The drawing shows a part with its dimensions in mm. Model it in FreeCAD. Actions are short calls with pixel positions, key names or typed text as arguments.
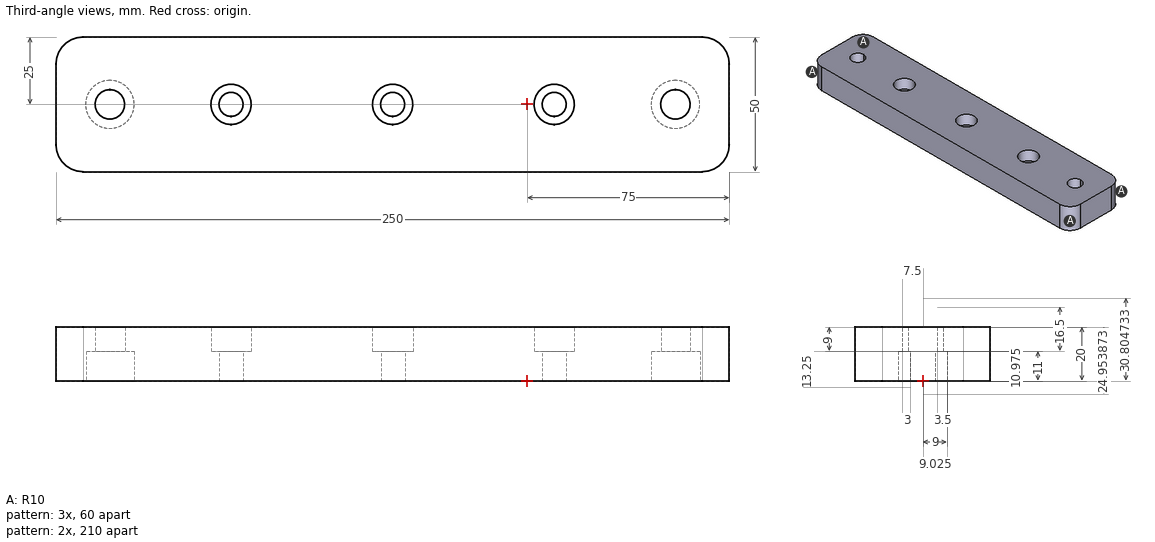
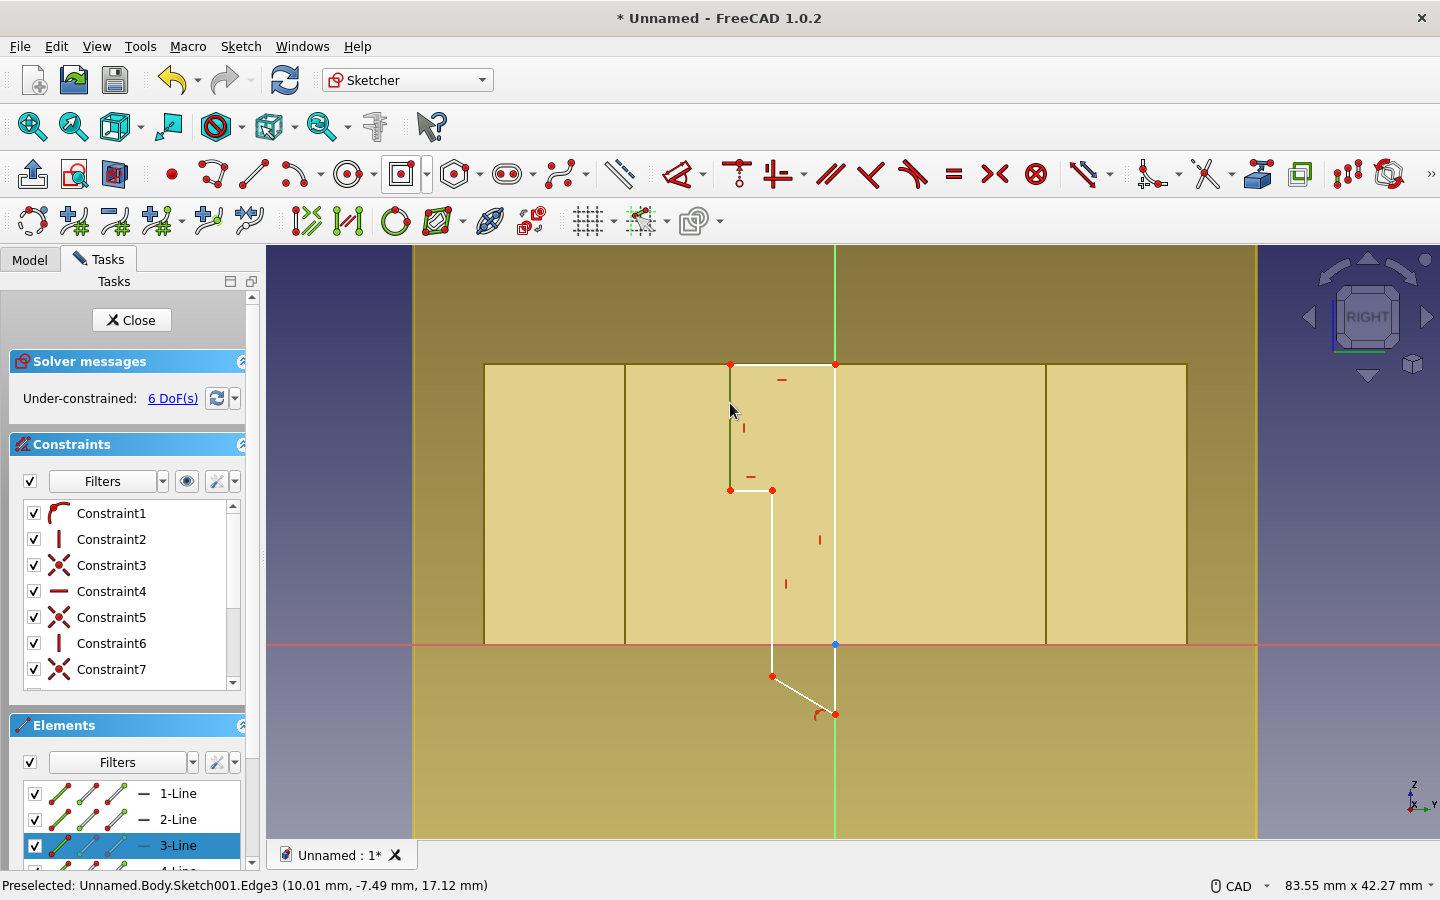
key(i)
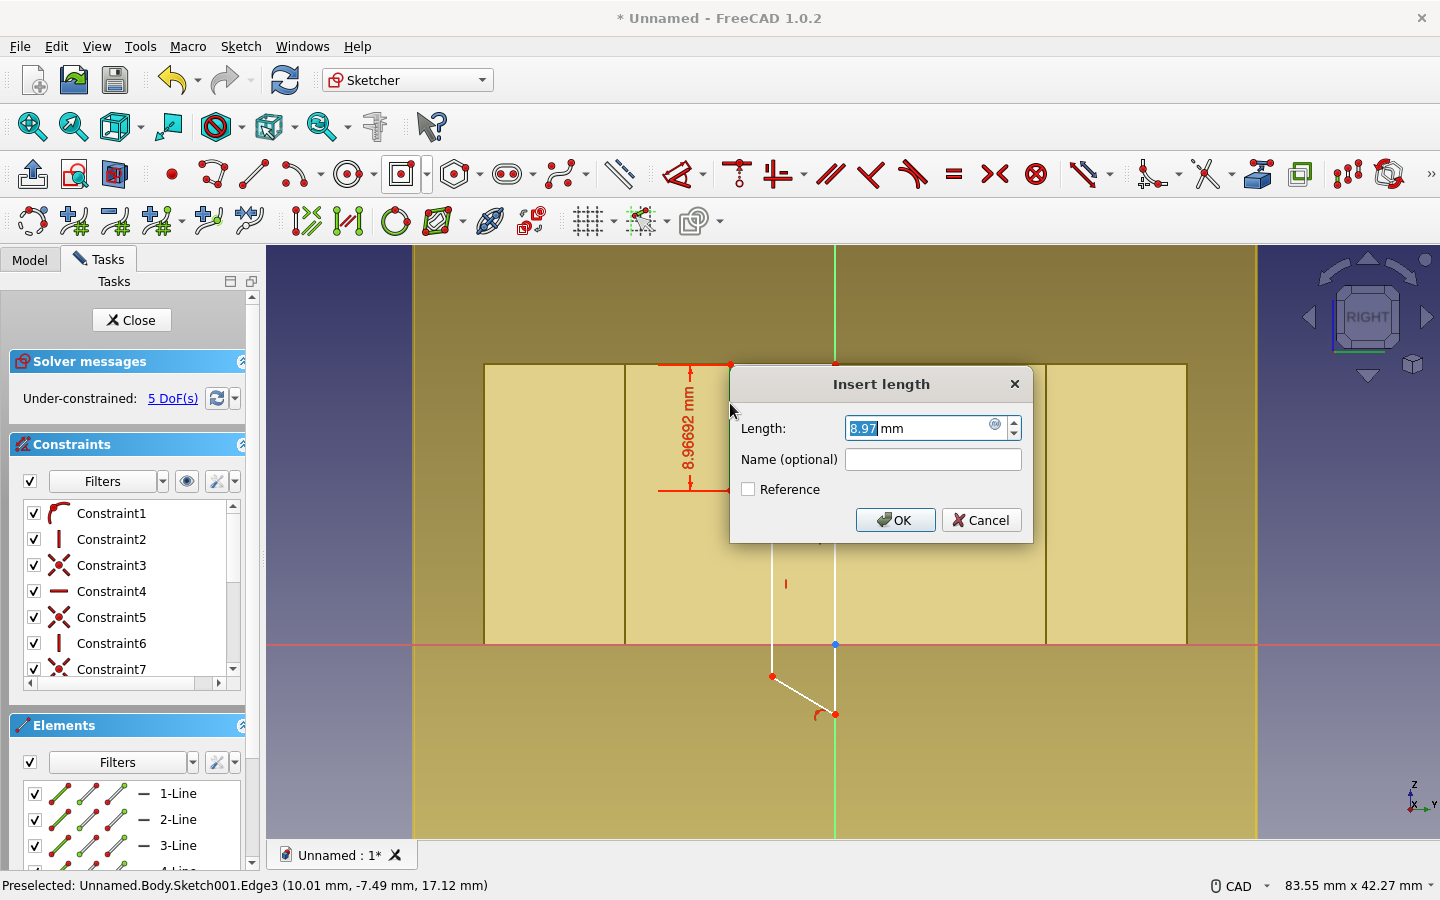
text(9)
key(Return)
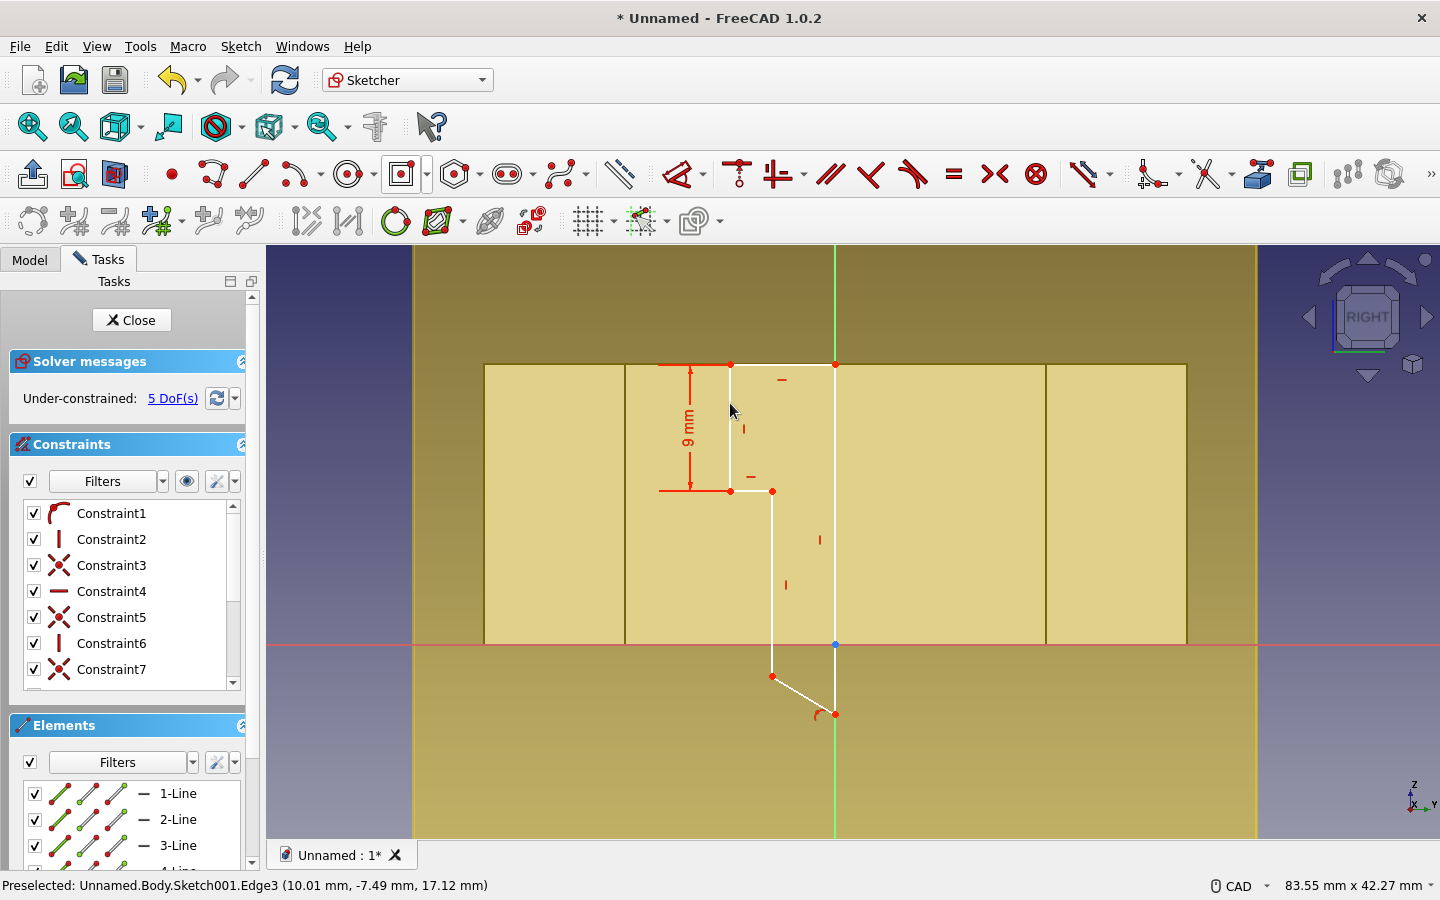
click(743, 491)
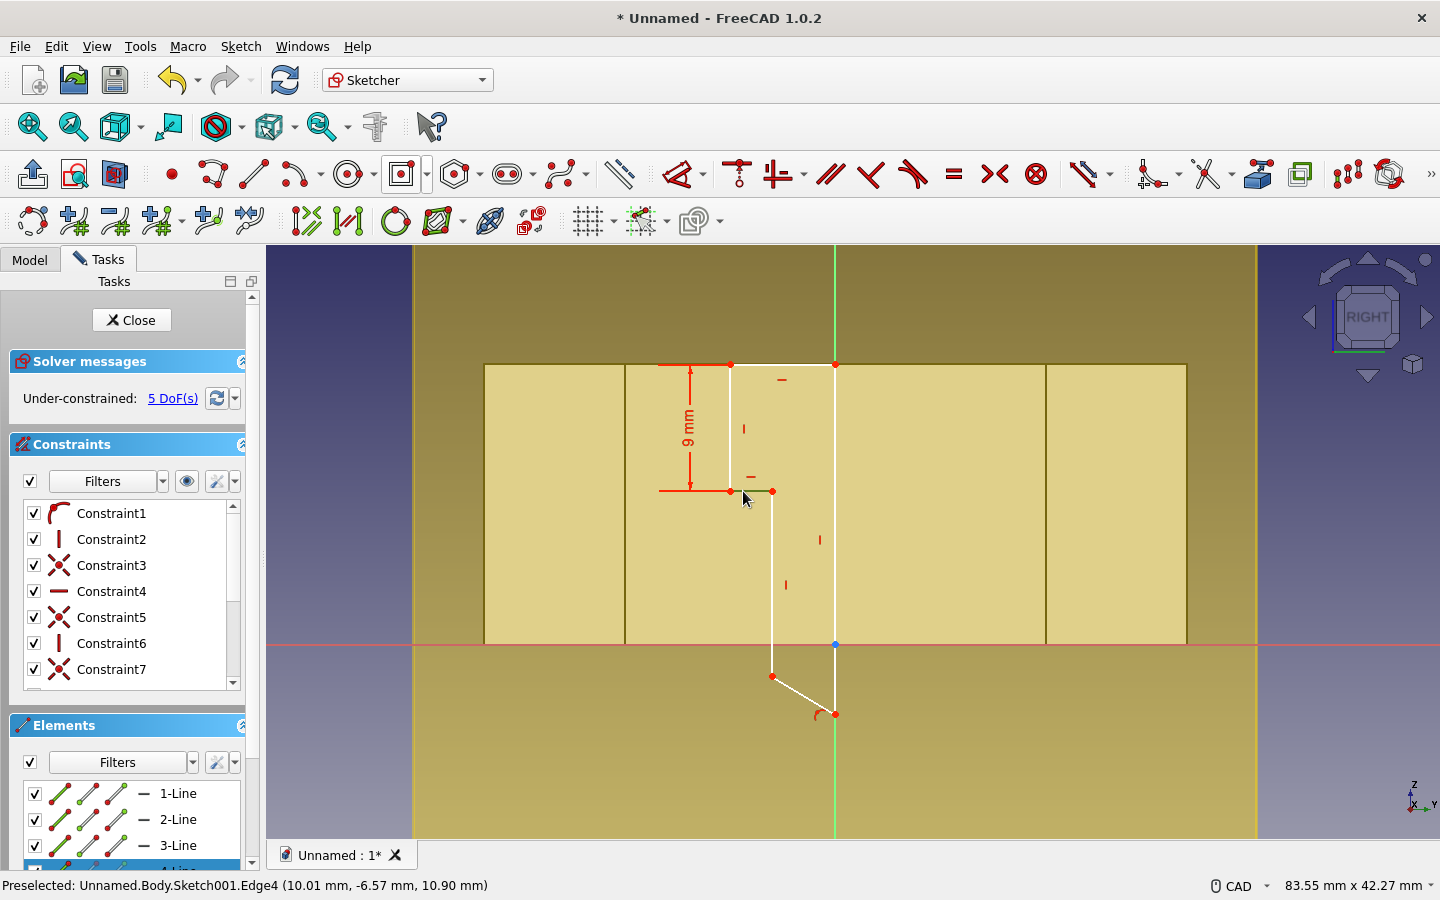
key(l)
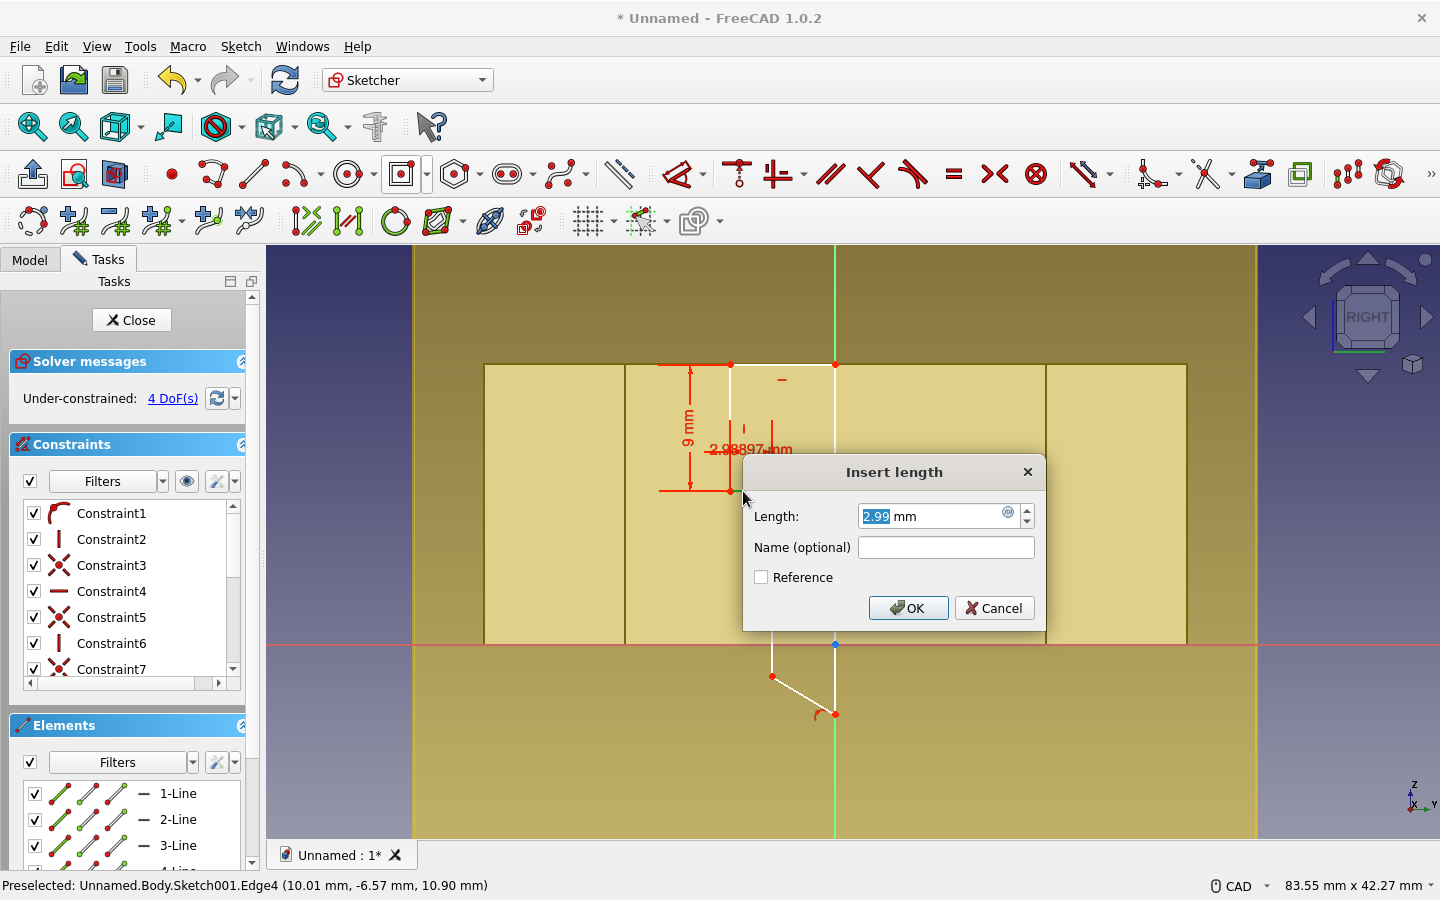
text(3)
key(Return)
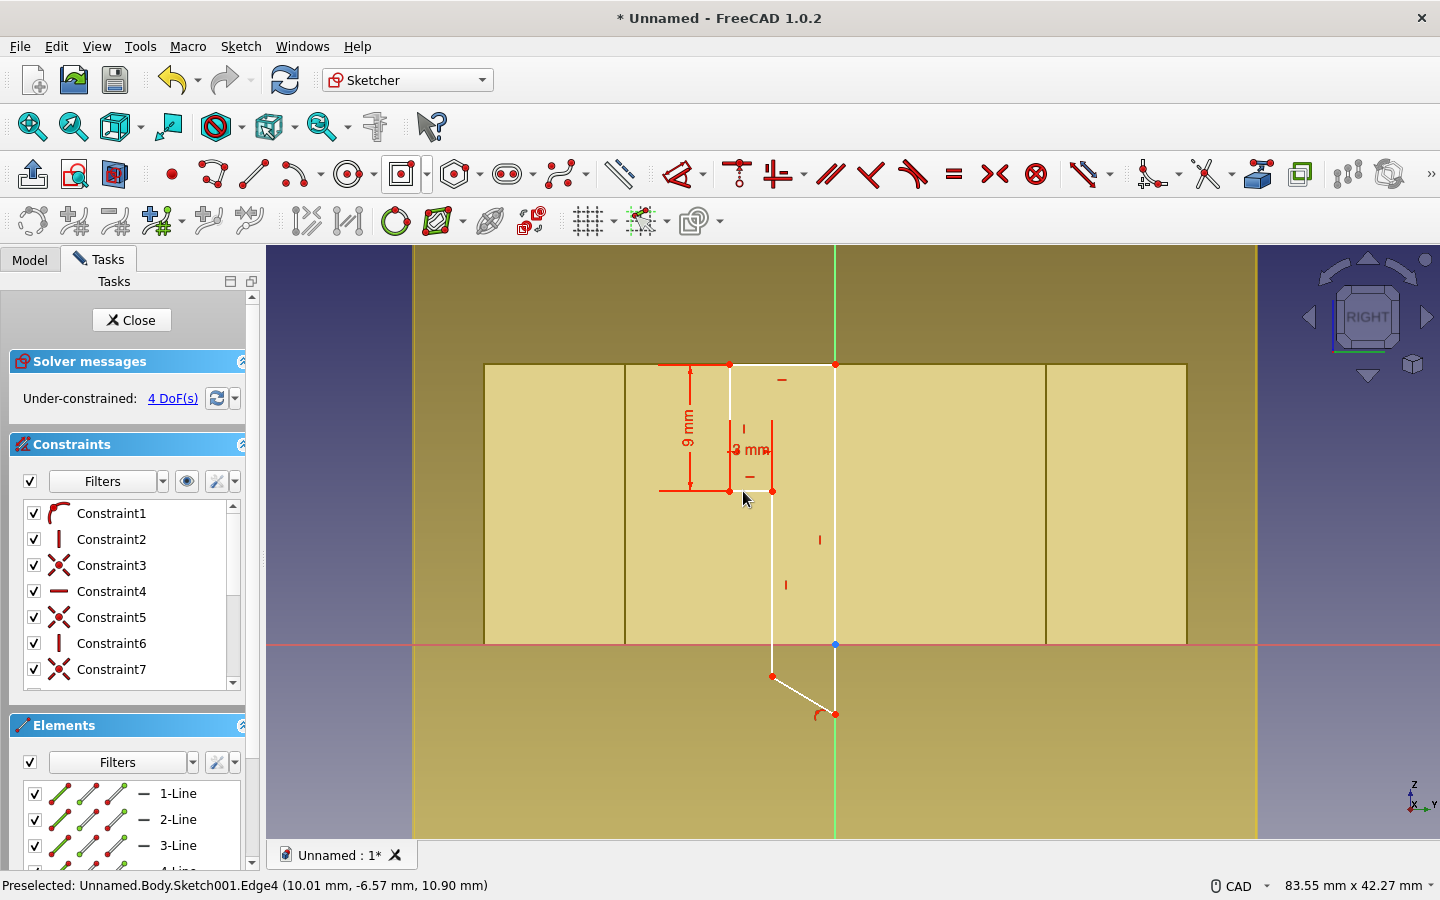
click(804, 365)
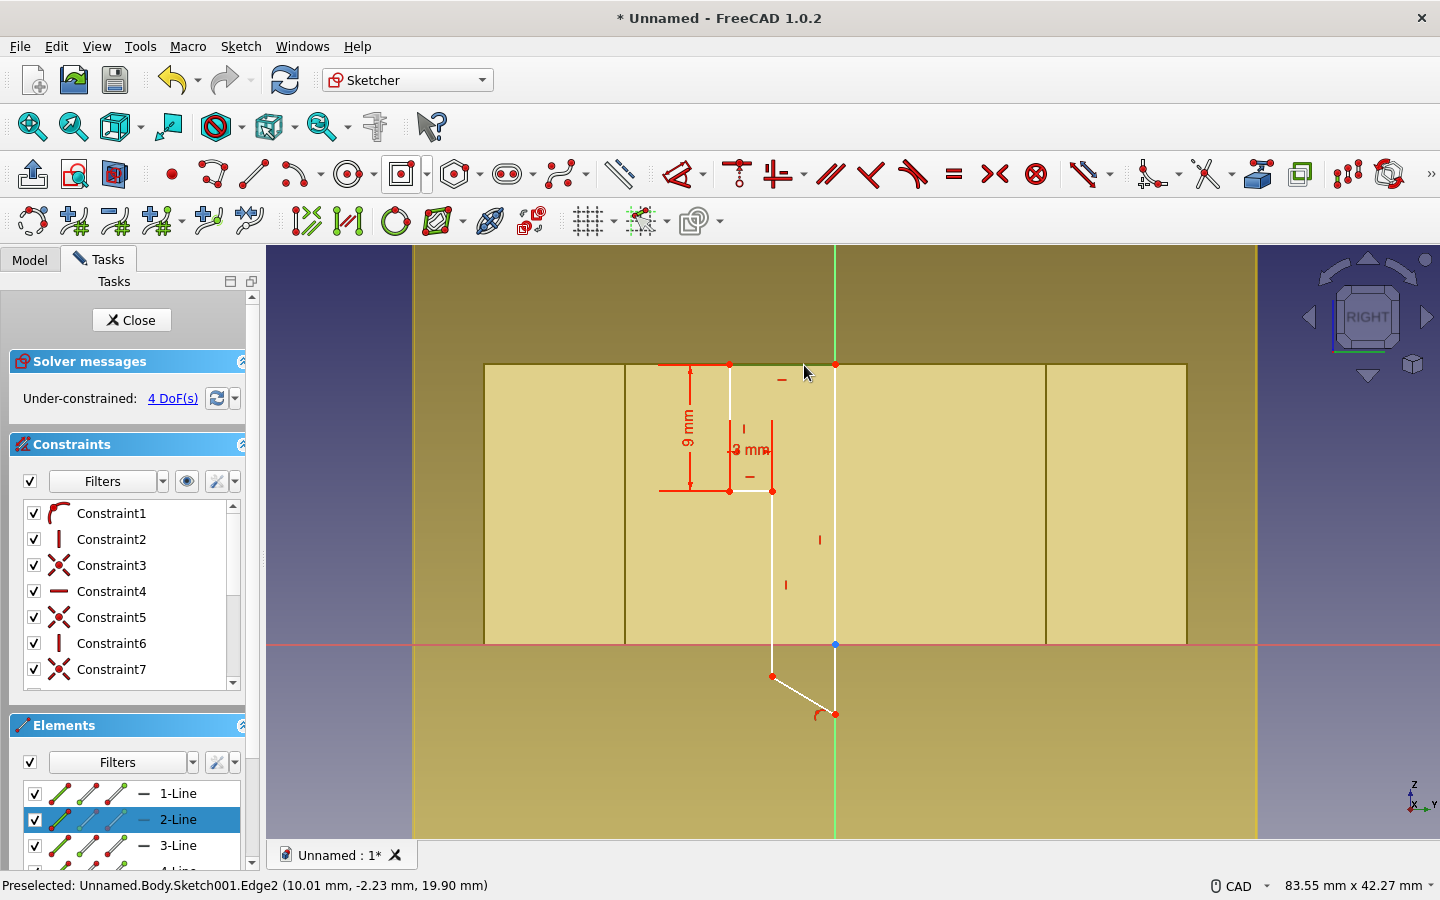
key(l)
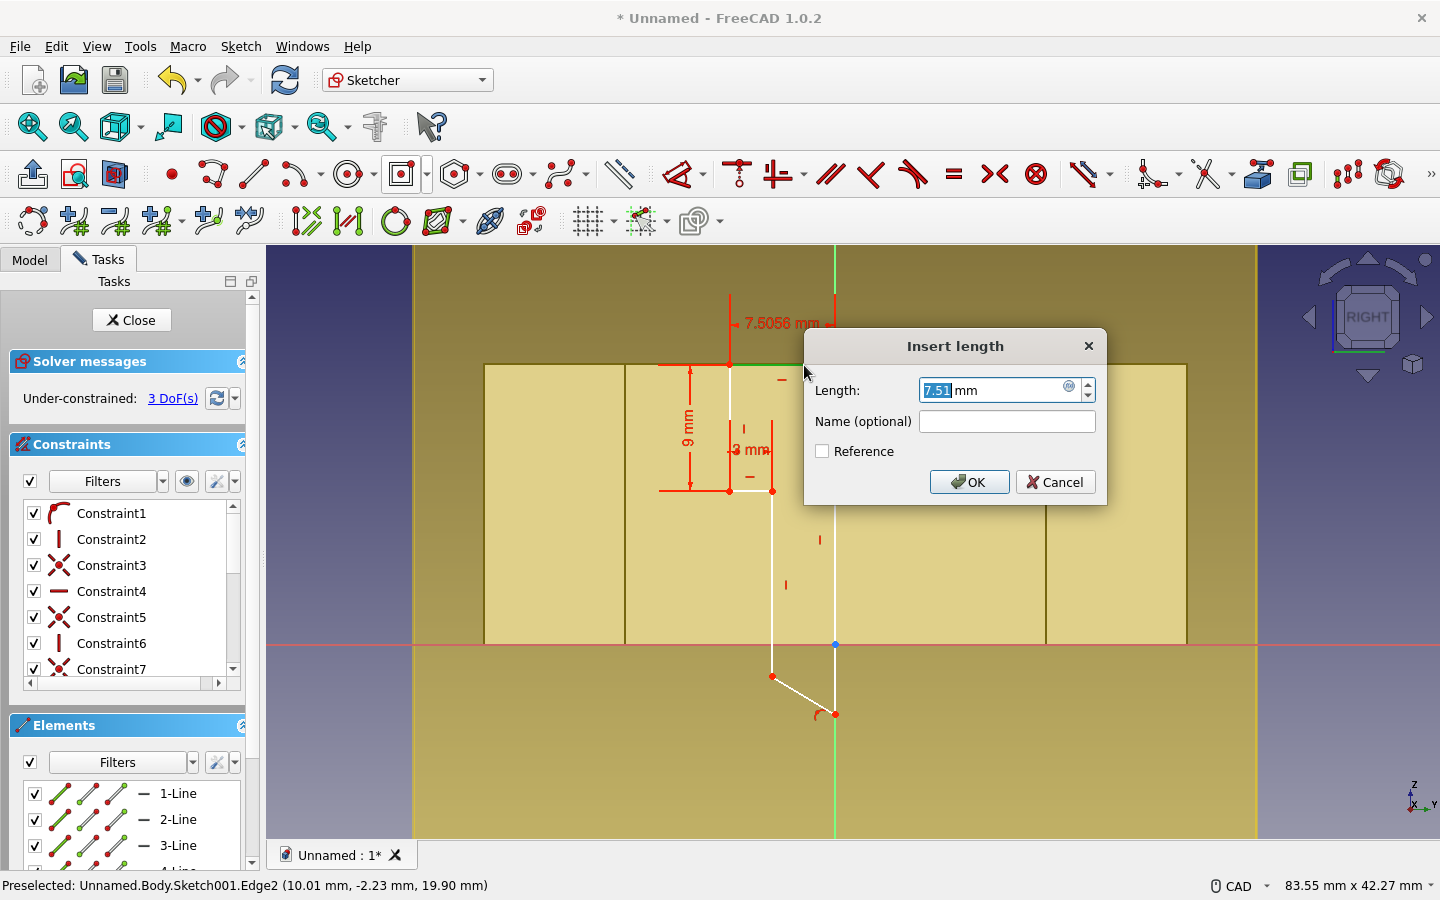
text(7.5)
key(Return)